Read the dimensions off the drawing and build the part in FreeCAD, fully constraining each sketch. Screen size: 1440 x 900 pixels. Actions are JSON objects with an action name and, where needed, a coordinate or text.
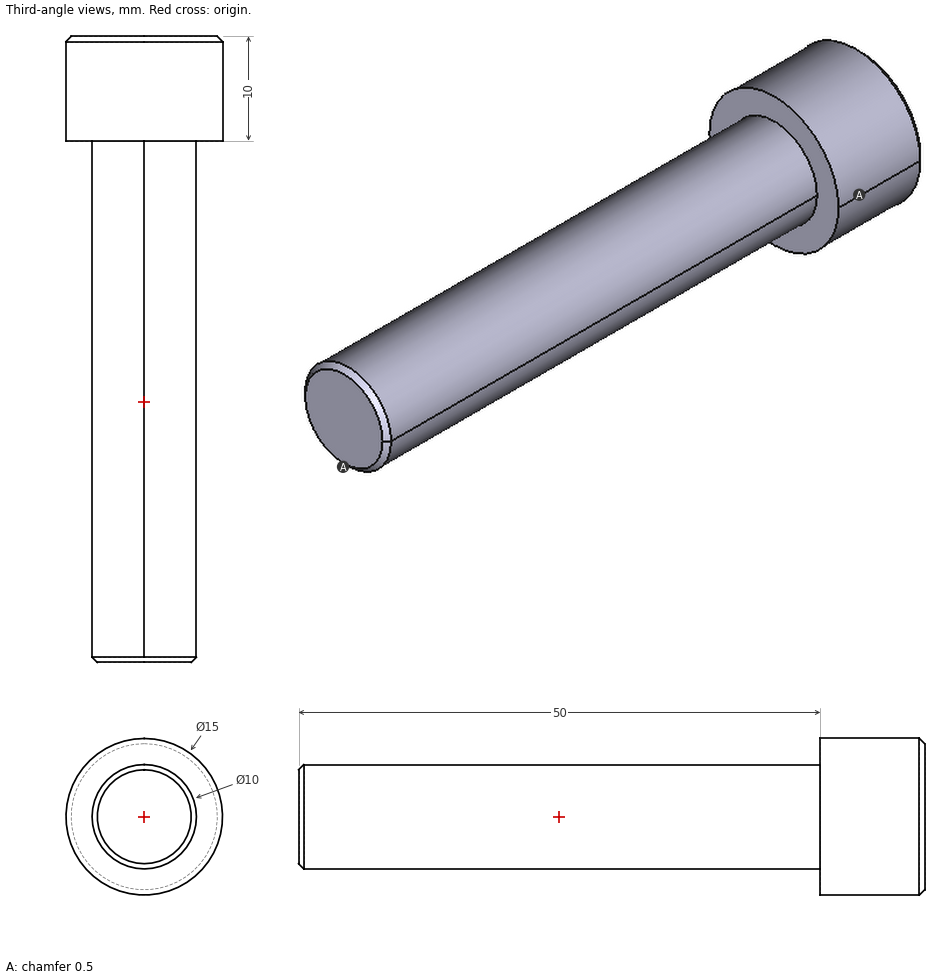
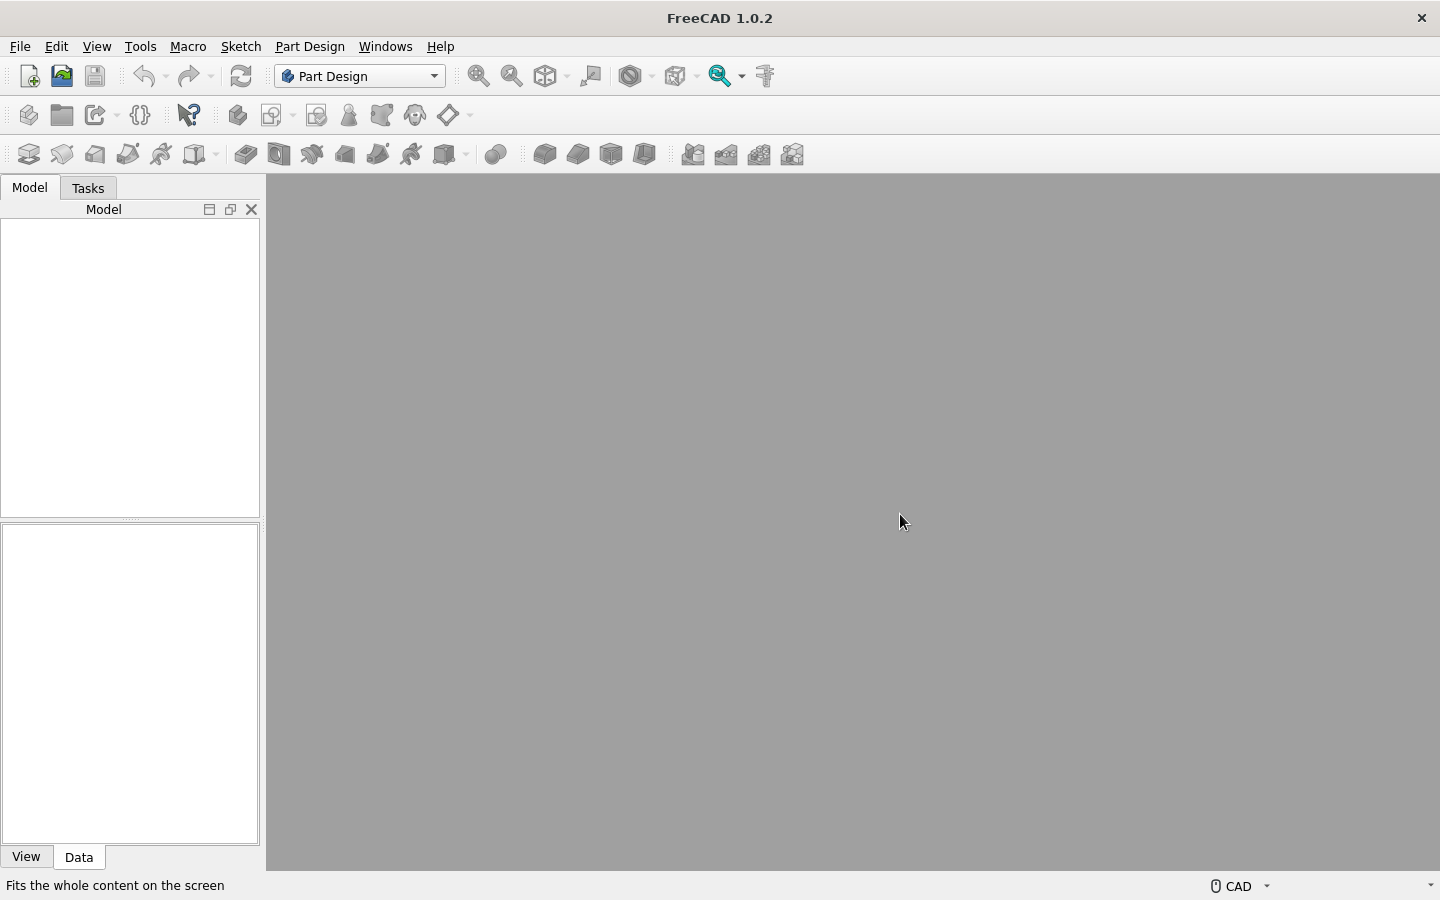
{"action": "key", "text": "ctrl+n"}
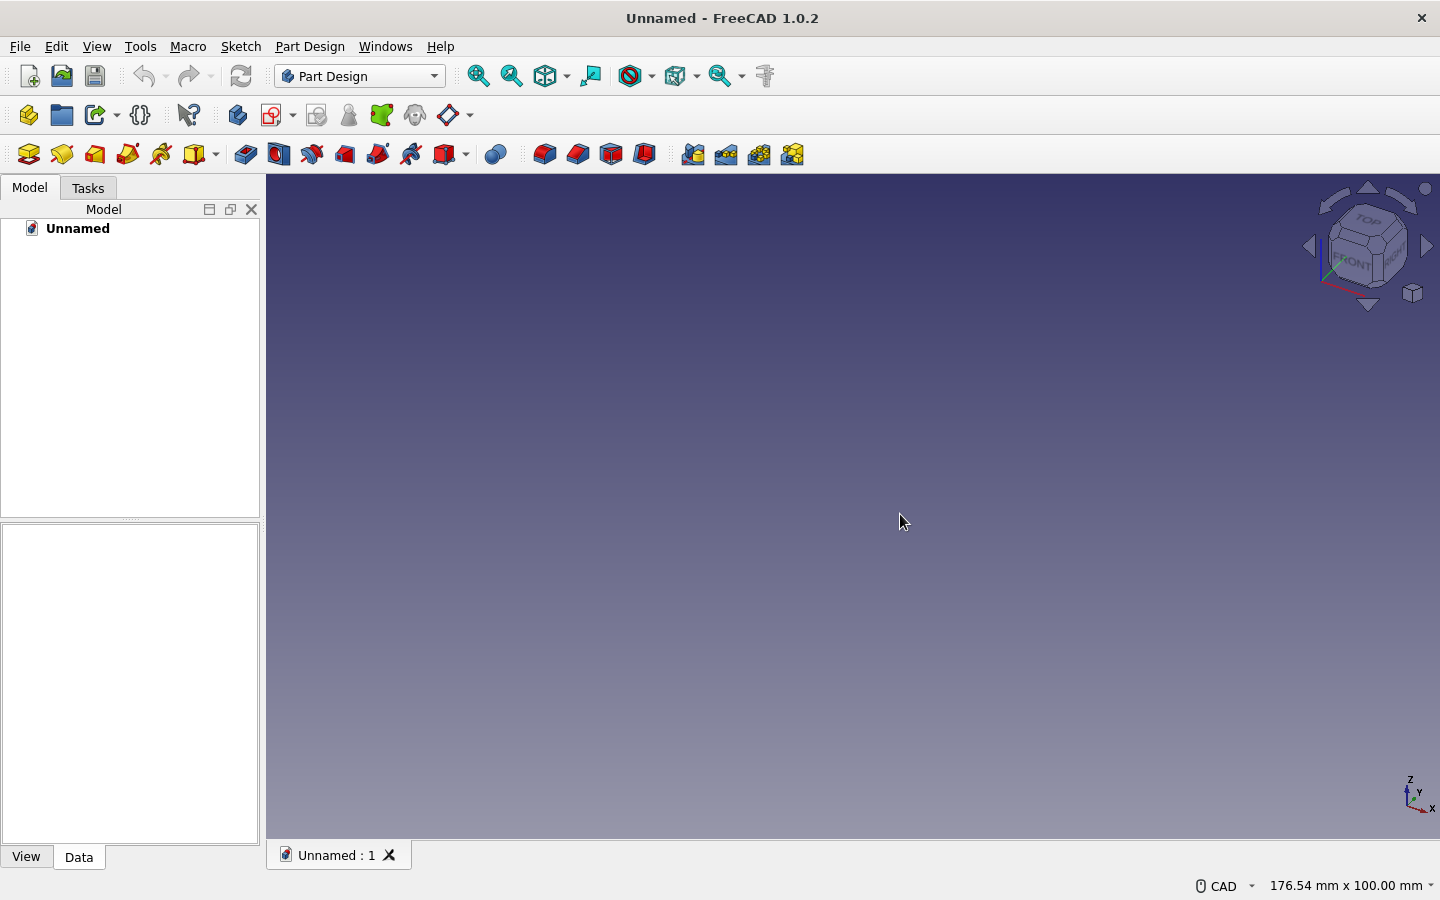
{"action": "left_click", "coordinate": [270, 116]}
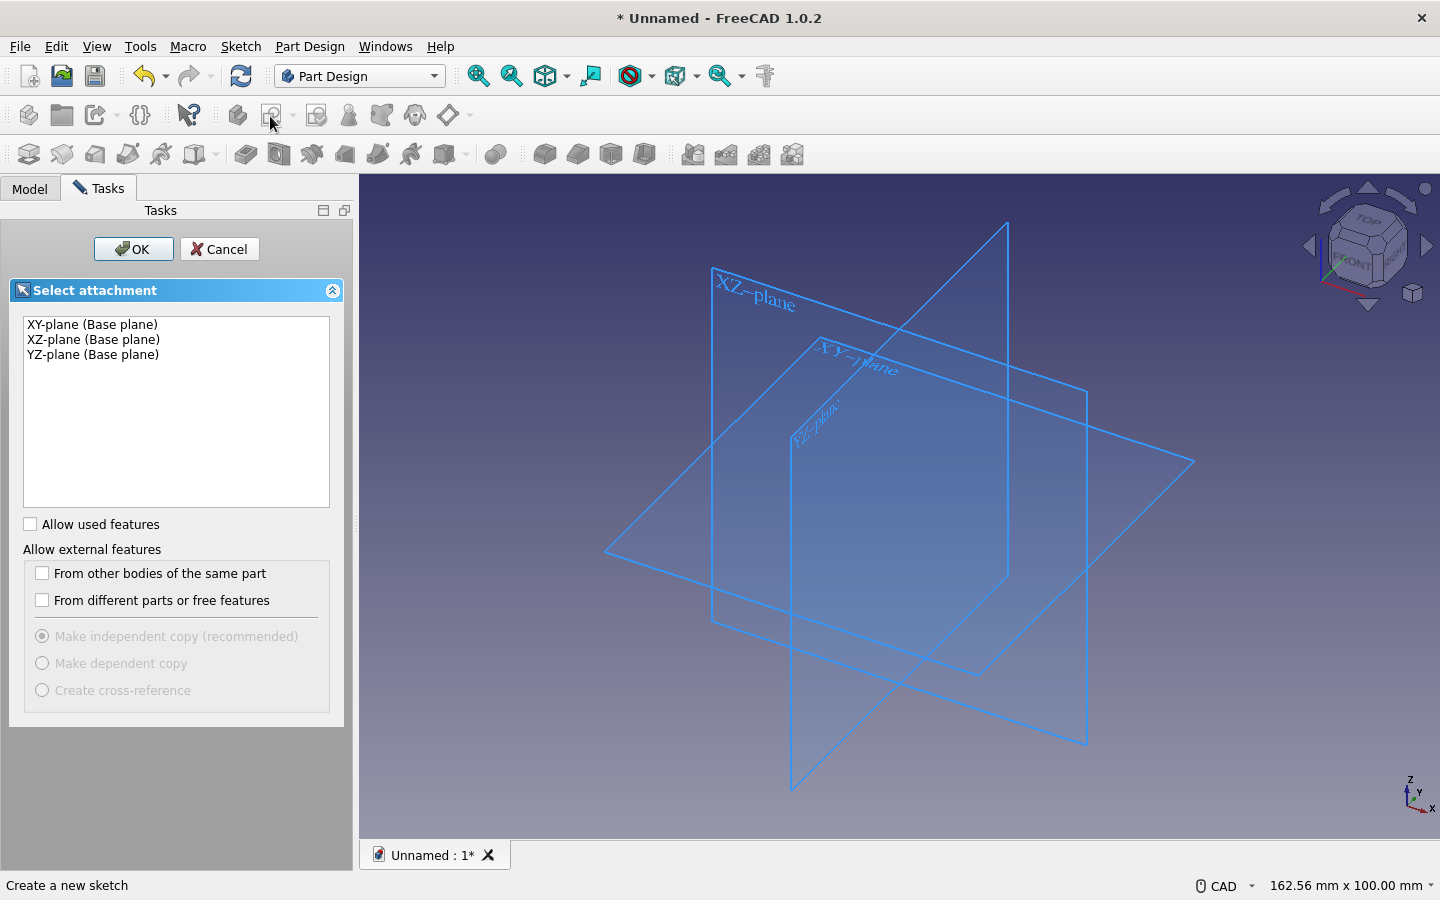
{"action": "left_click", "coordinate": [84, 340]}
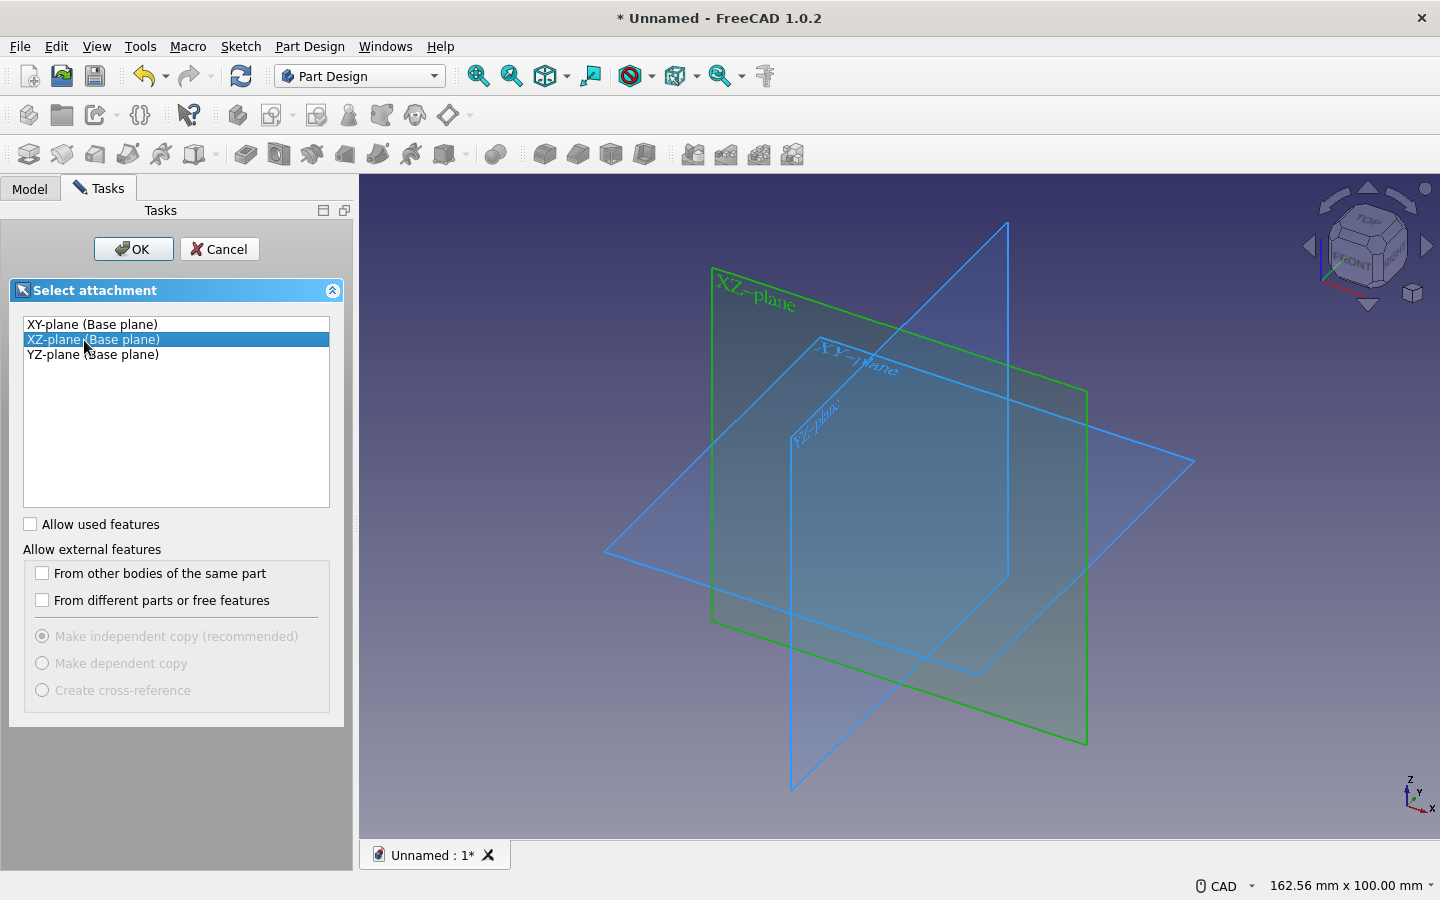
{"action": "left_click", "coordinate": [134, 249]}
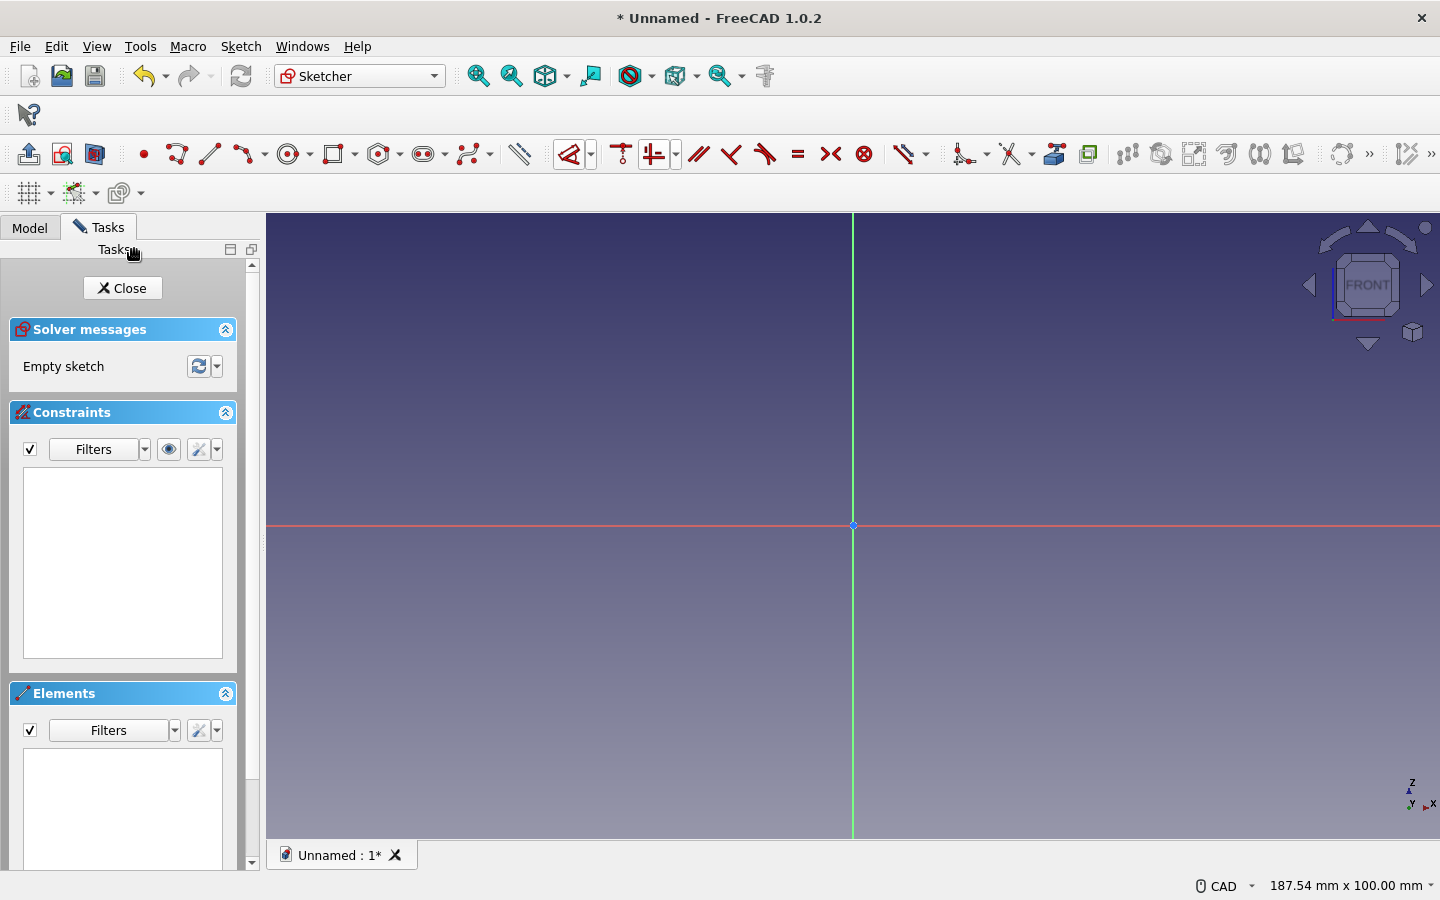
{"action": "scroll", "coordinate": [867, 526], "scroll_direction": "up", "scroll_amount": 9}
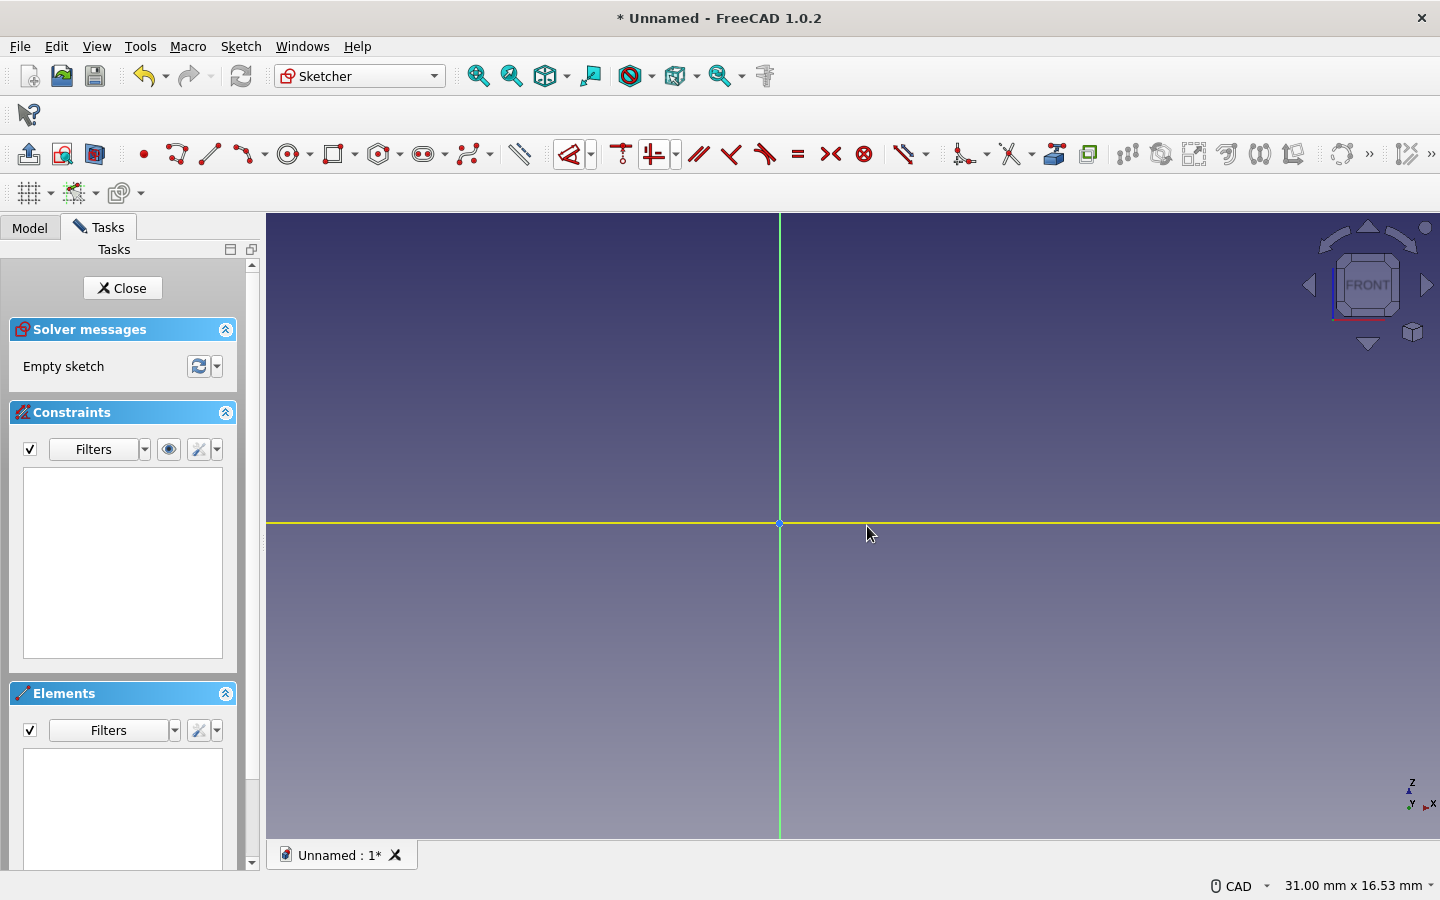
{"action": "left_click", "coordinate": [288, 154]}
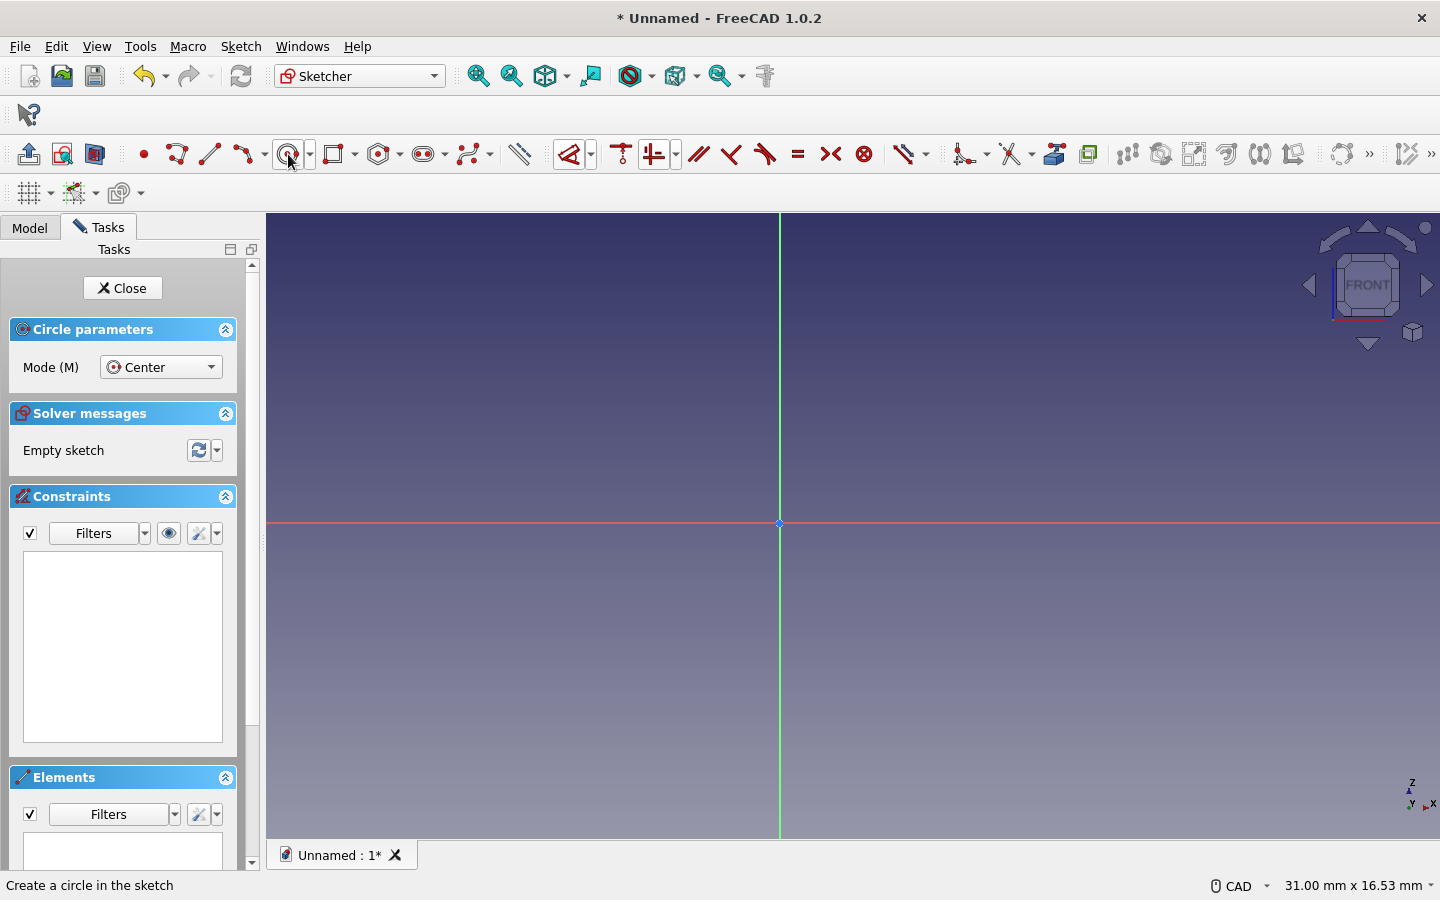
{"action": "left_click", "coordinate": [780, 523]}
{"action": "mouse_move", "coordinate": [914, 390]}